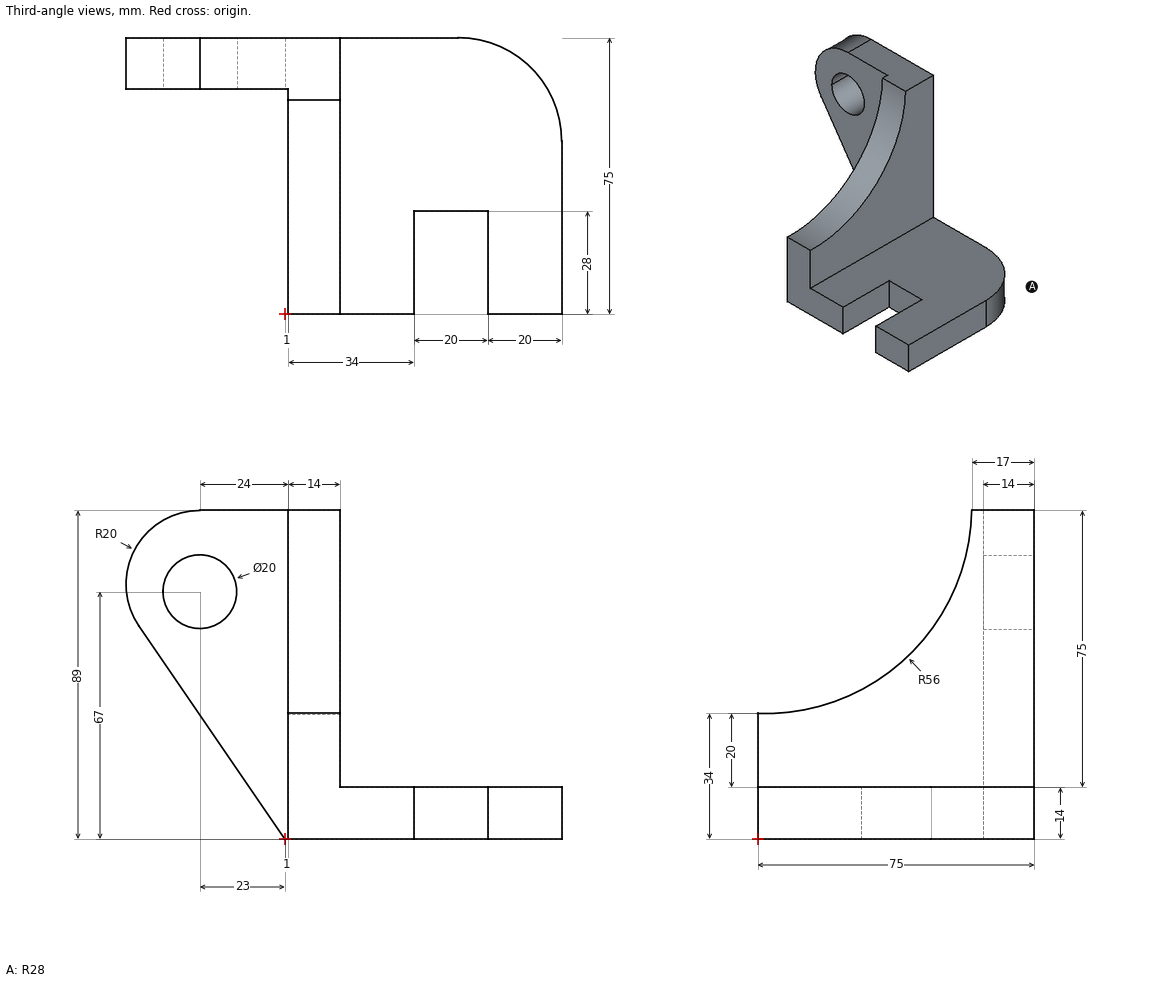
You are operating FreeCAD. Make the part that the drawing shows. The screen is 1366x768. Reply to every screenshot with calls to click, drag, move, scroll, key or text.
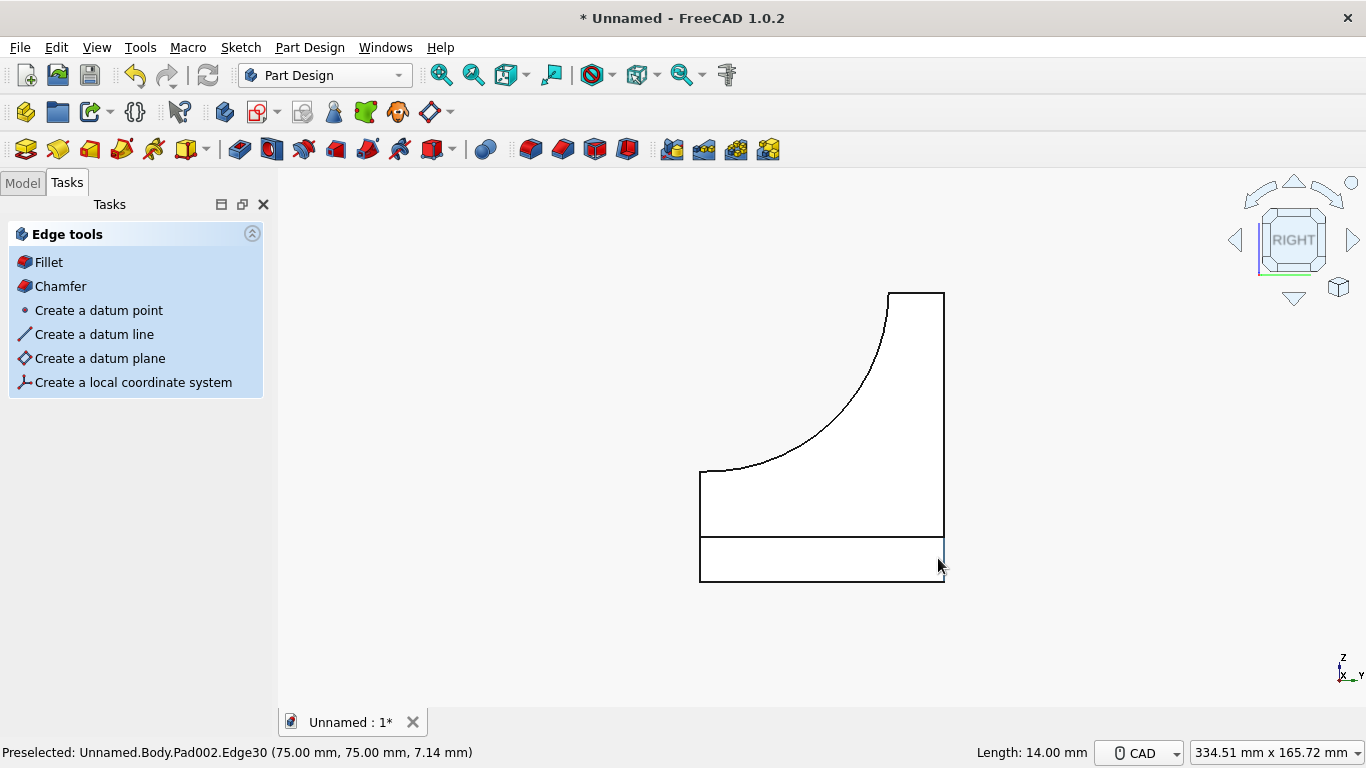
click(532, 150)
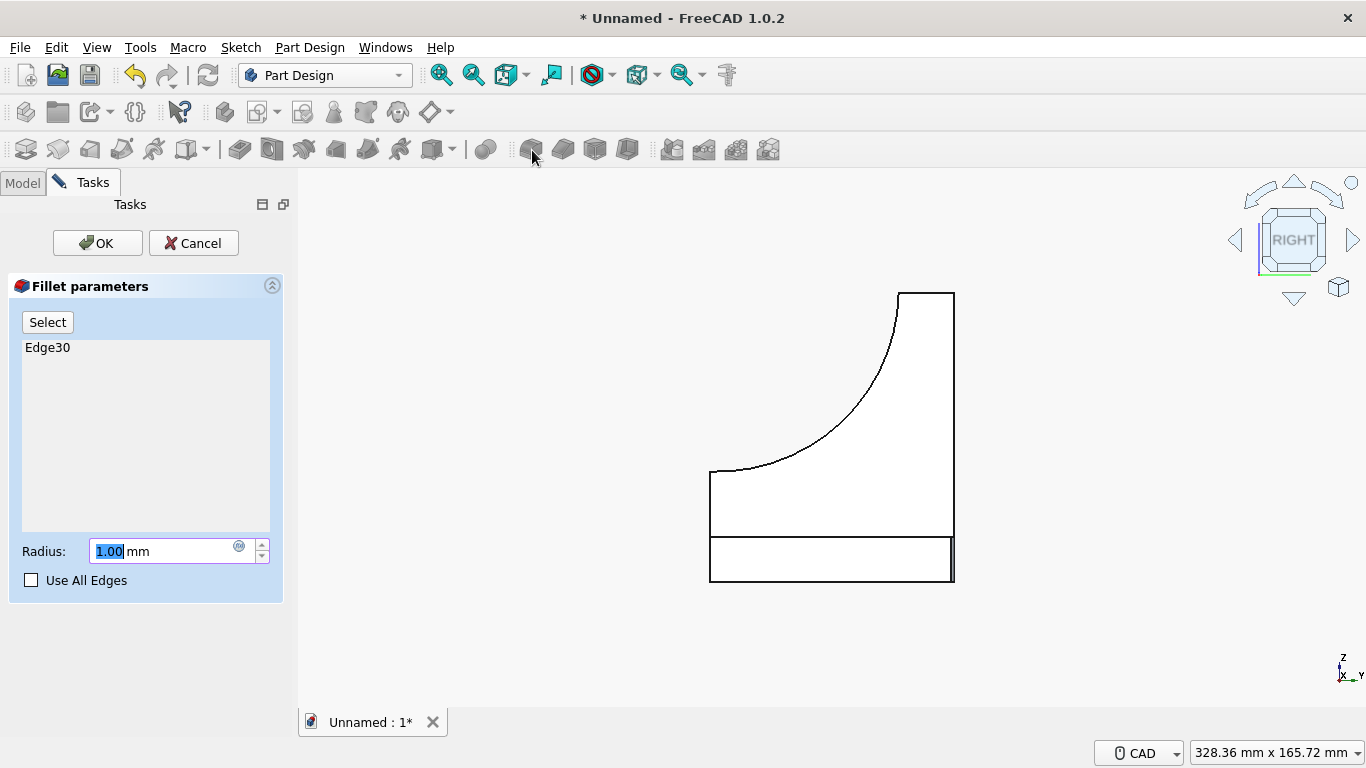
text(28)
key(Tab)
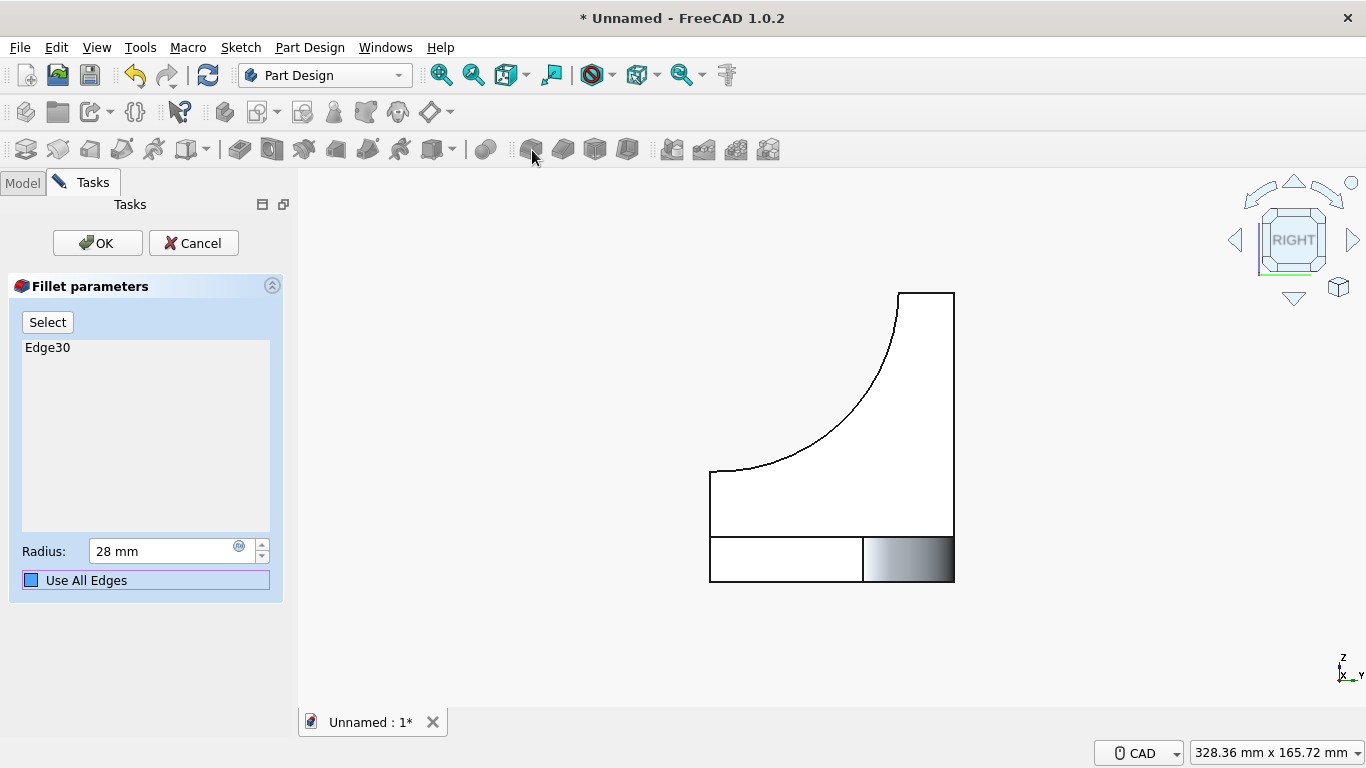
click(98, 243)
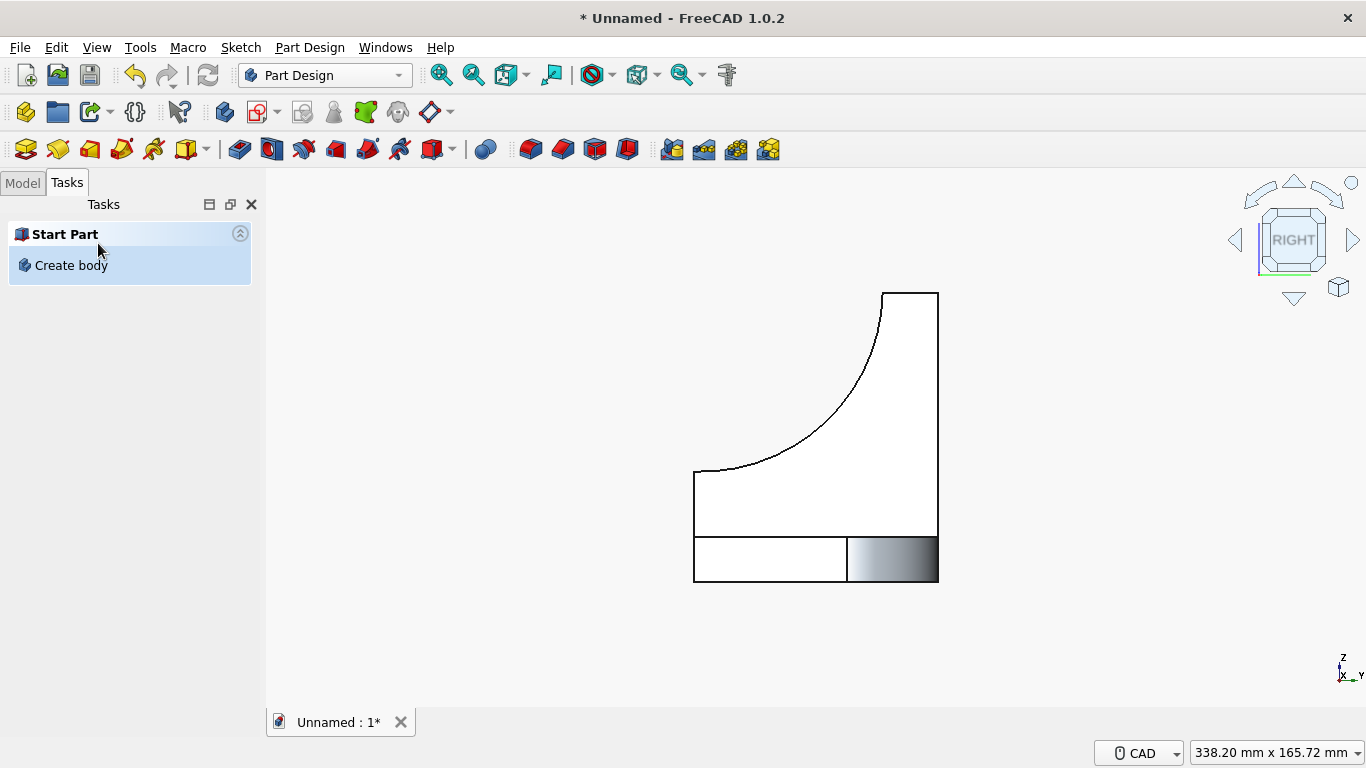
key(0)